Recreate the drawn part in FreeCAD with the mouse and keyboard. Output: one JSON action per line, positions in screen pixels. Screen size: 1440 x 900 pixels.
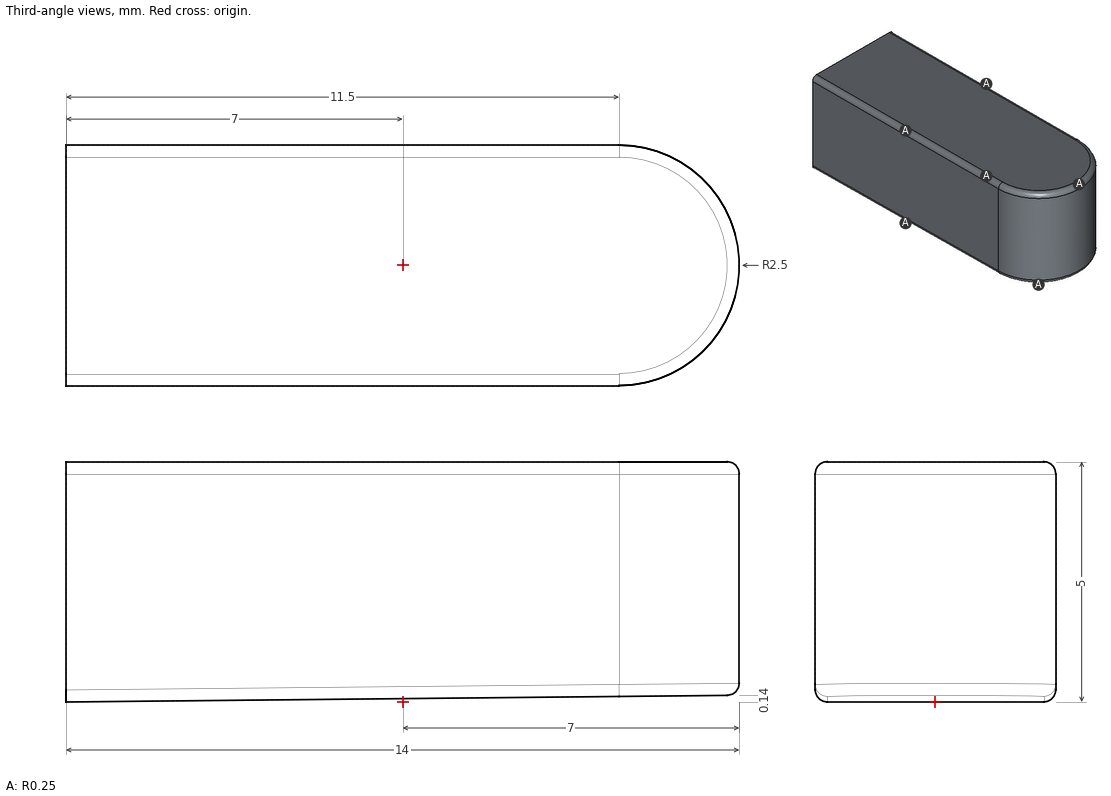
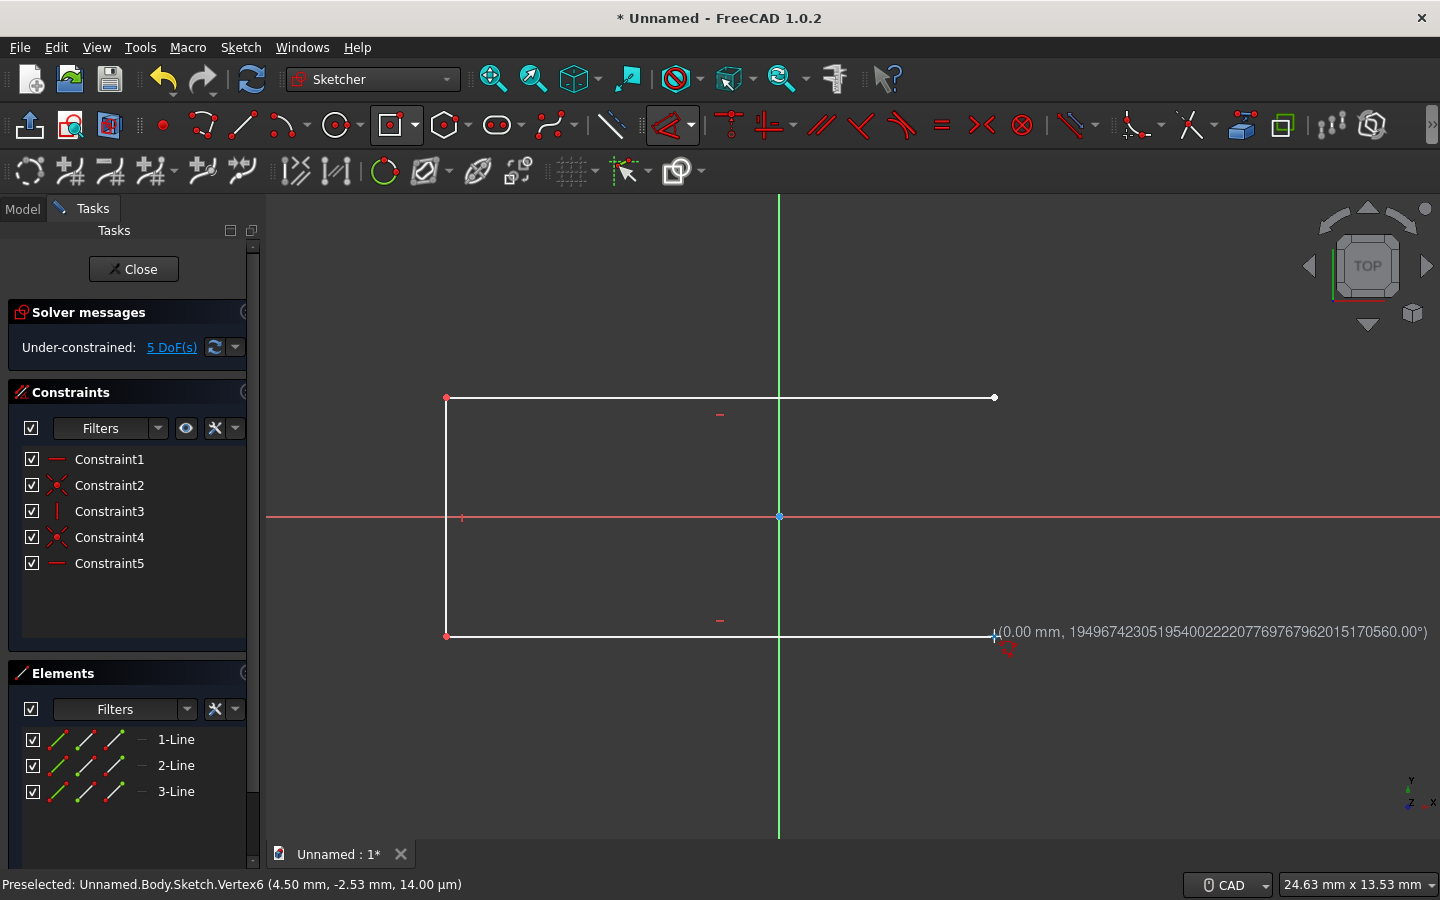
{"action": "key", "text": "g 3 a"}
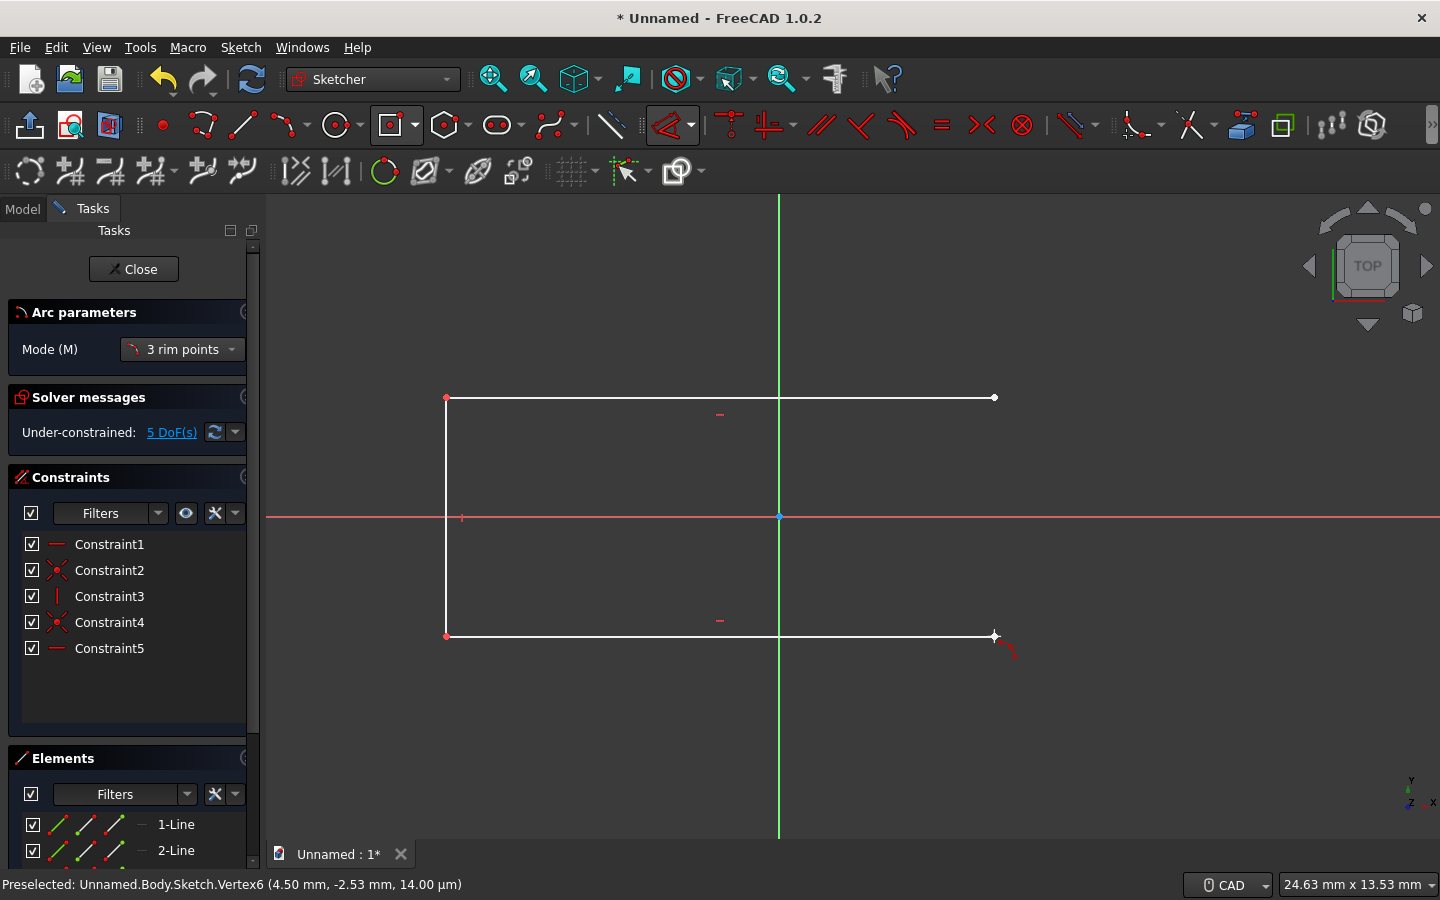
{"action": "left_click", "coordinate": [994, 637]}
{"action": "left_click", "coordinate": [994, 398]}
{"action": "left_click", "coordinate": [1107, 553]}
{"action": "key", "text": "Escape"}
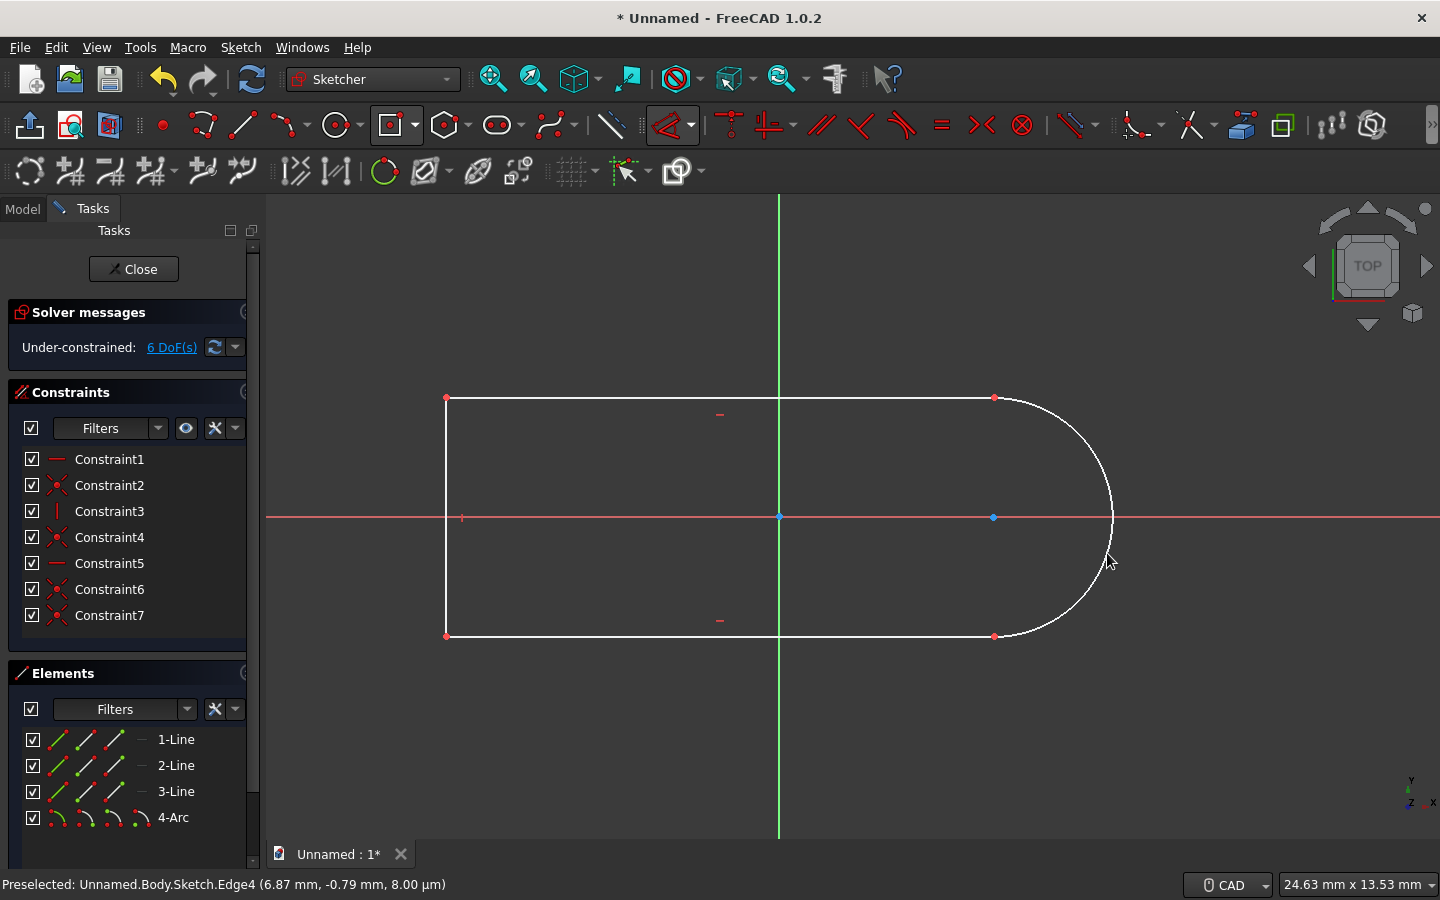
{"action": "left_click", "coordinate": [830, 398]}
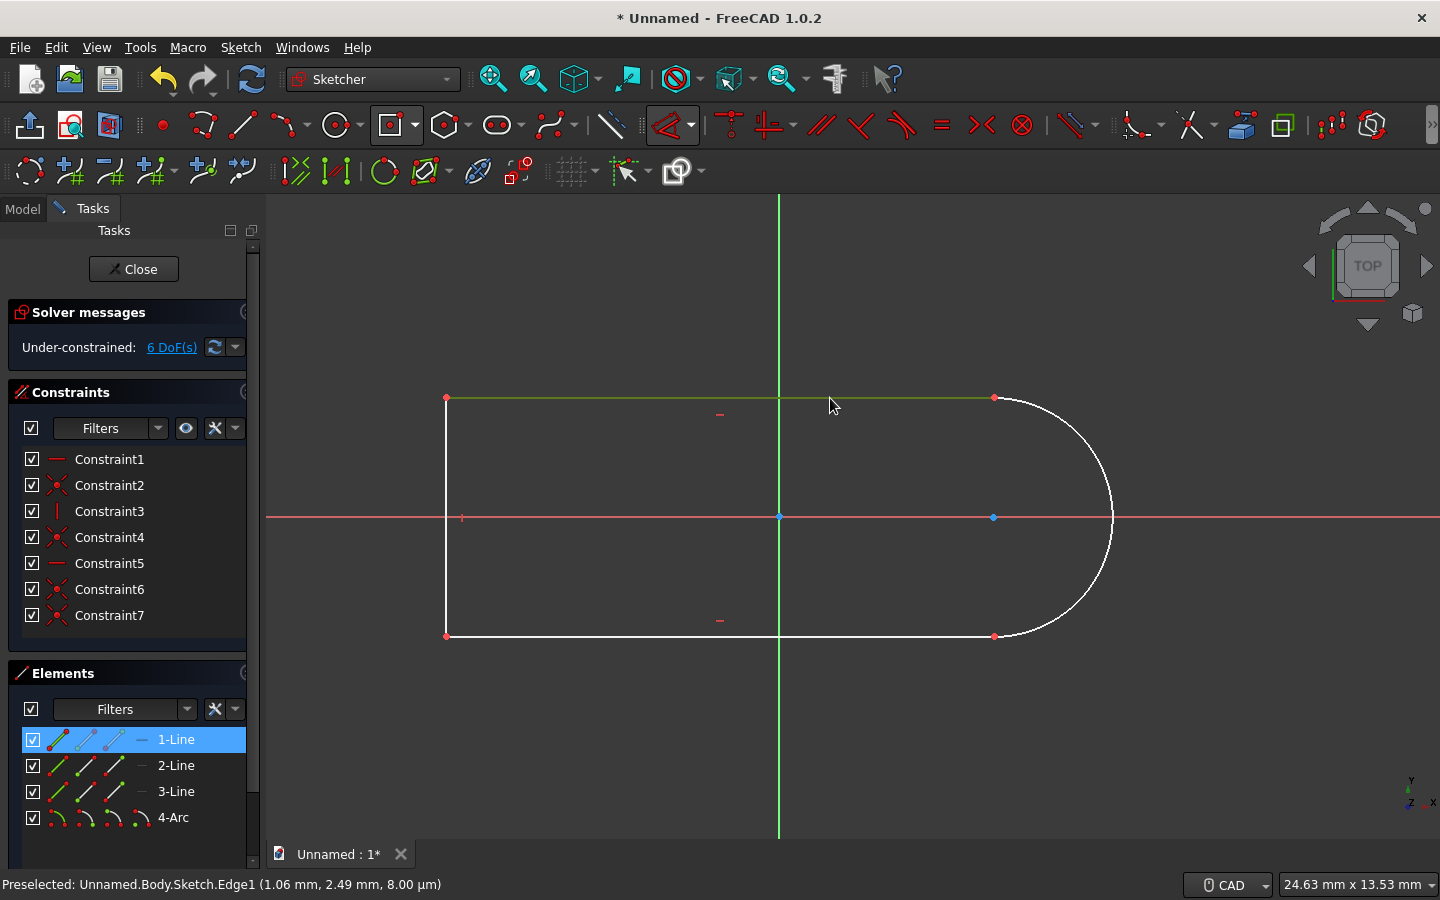
{"action": "left_click", "coordinate": [1090, 587]}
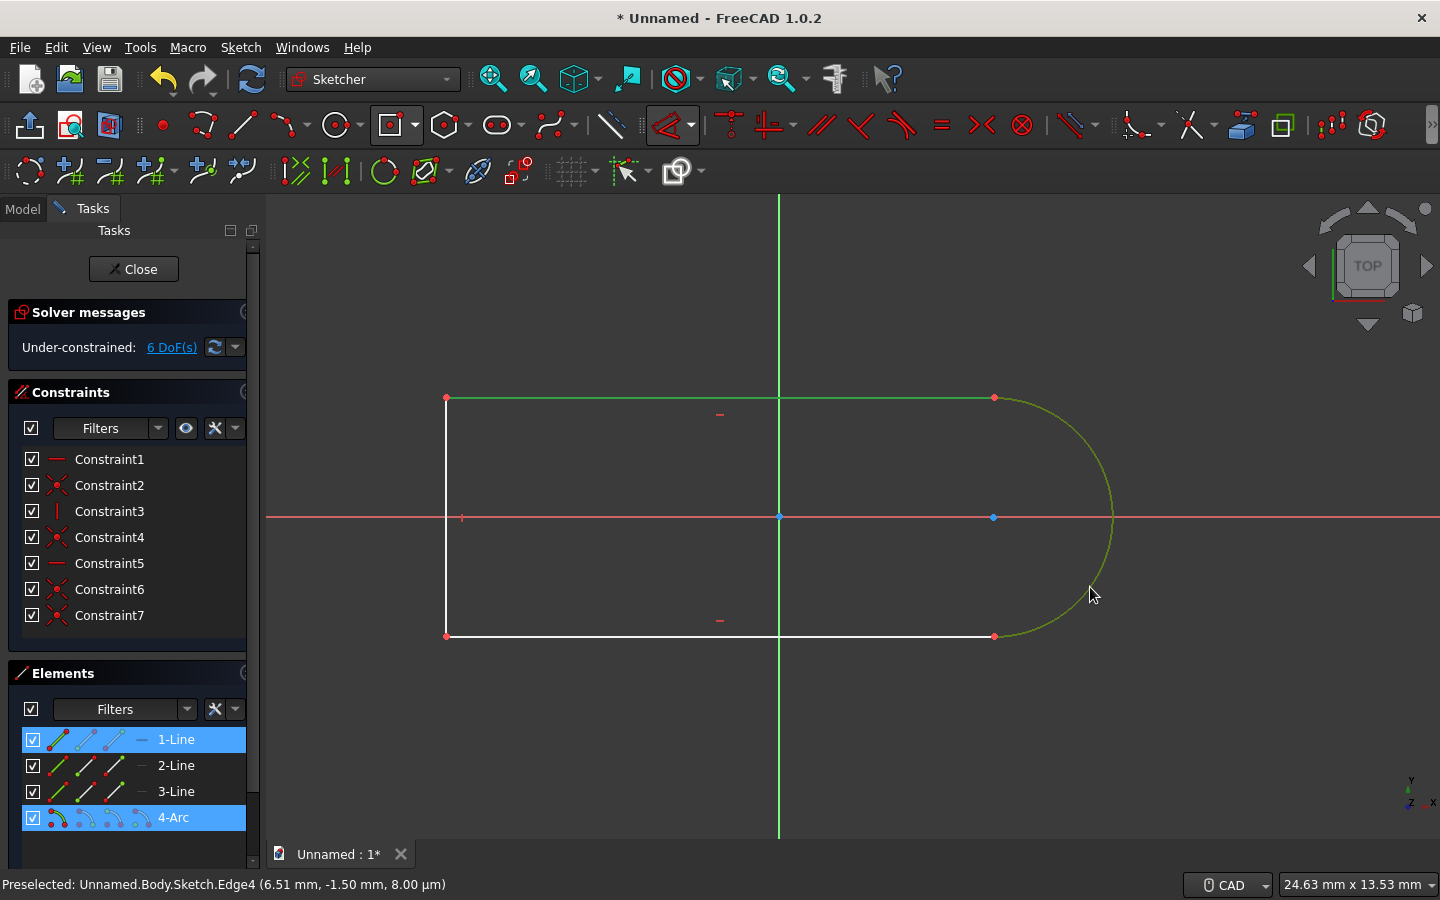
{"action": "key", "text": "t"}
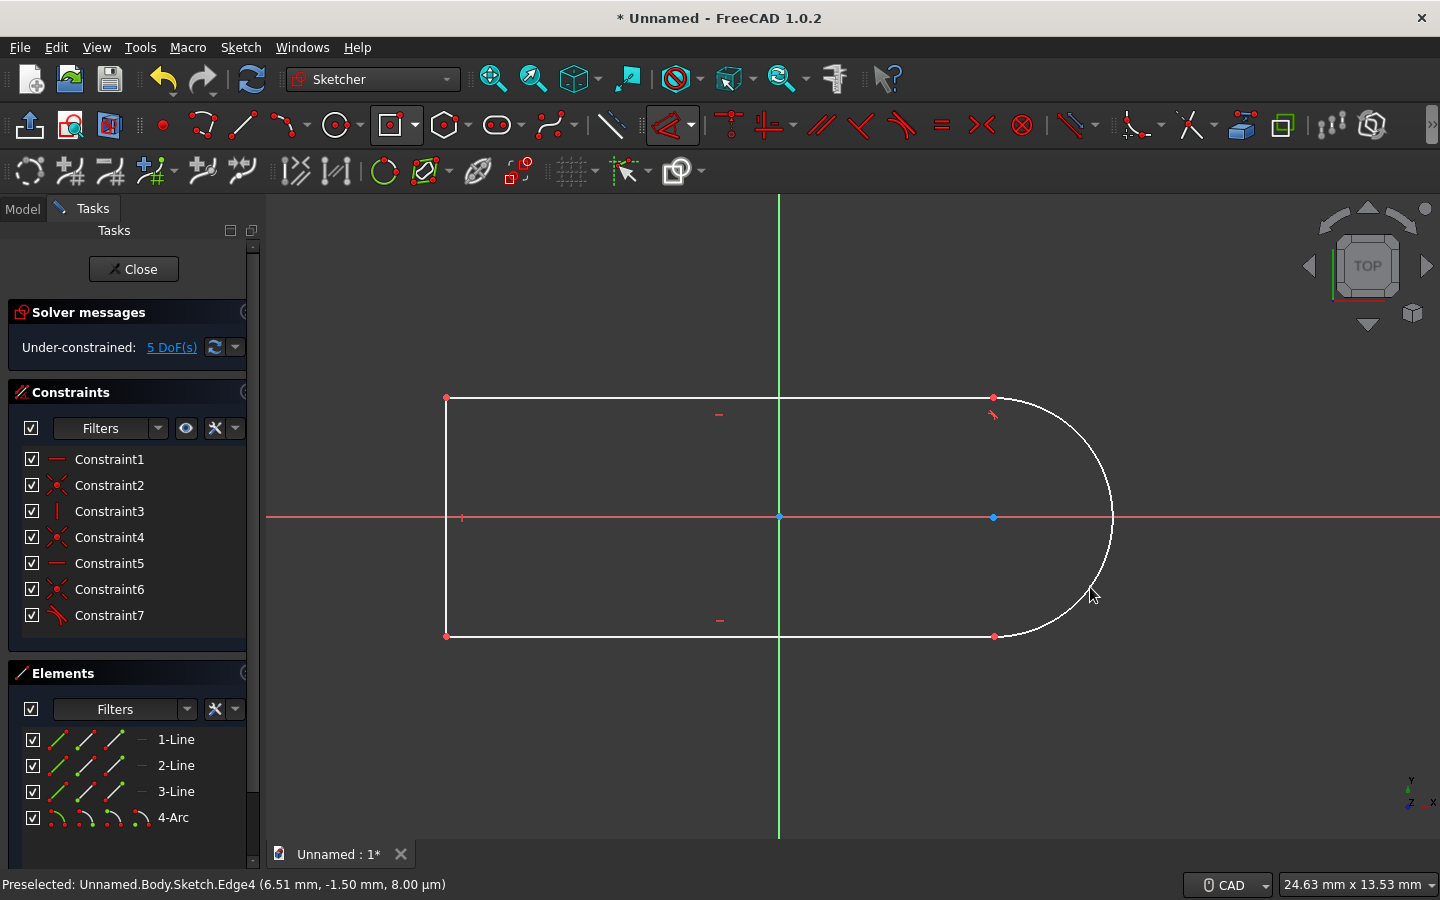
{"action": "left_click", "coordinate": [610, 637]}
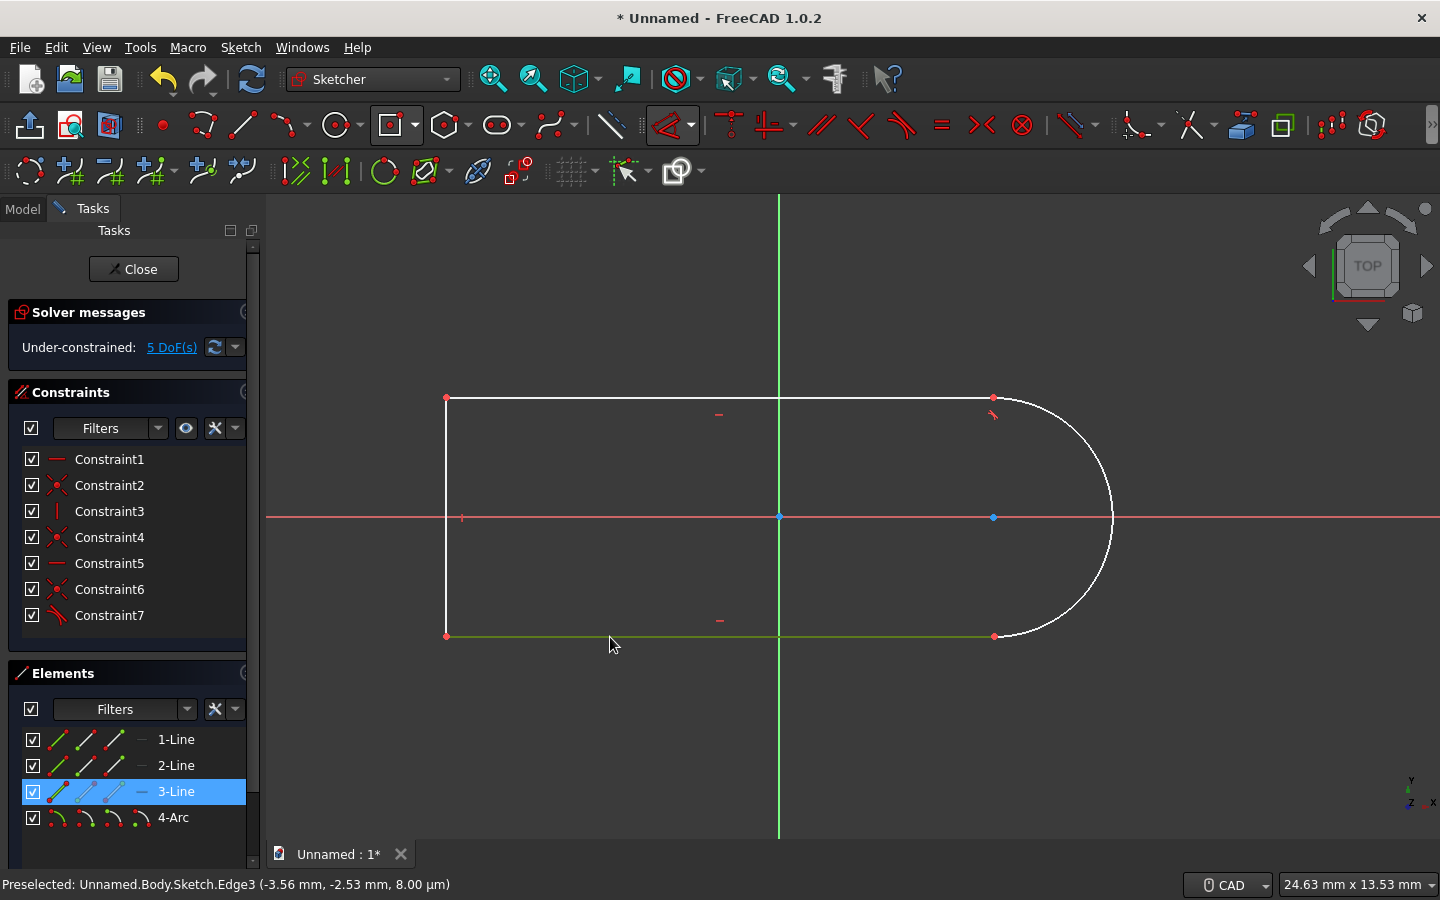
{"action": "left_click", "coordinate": [1090, 587]}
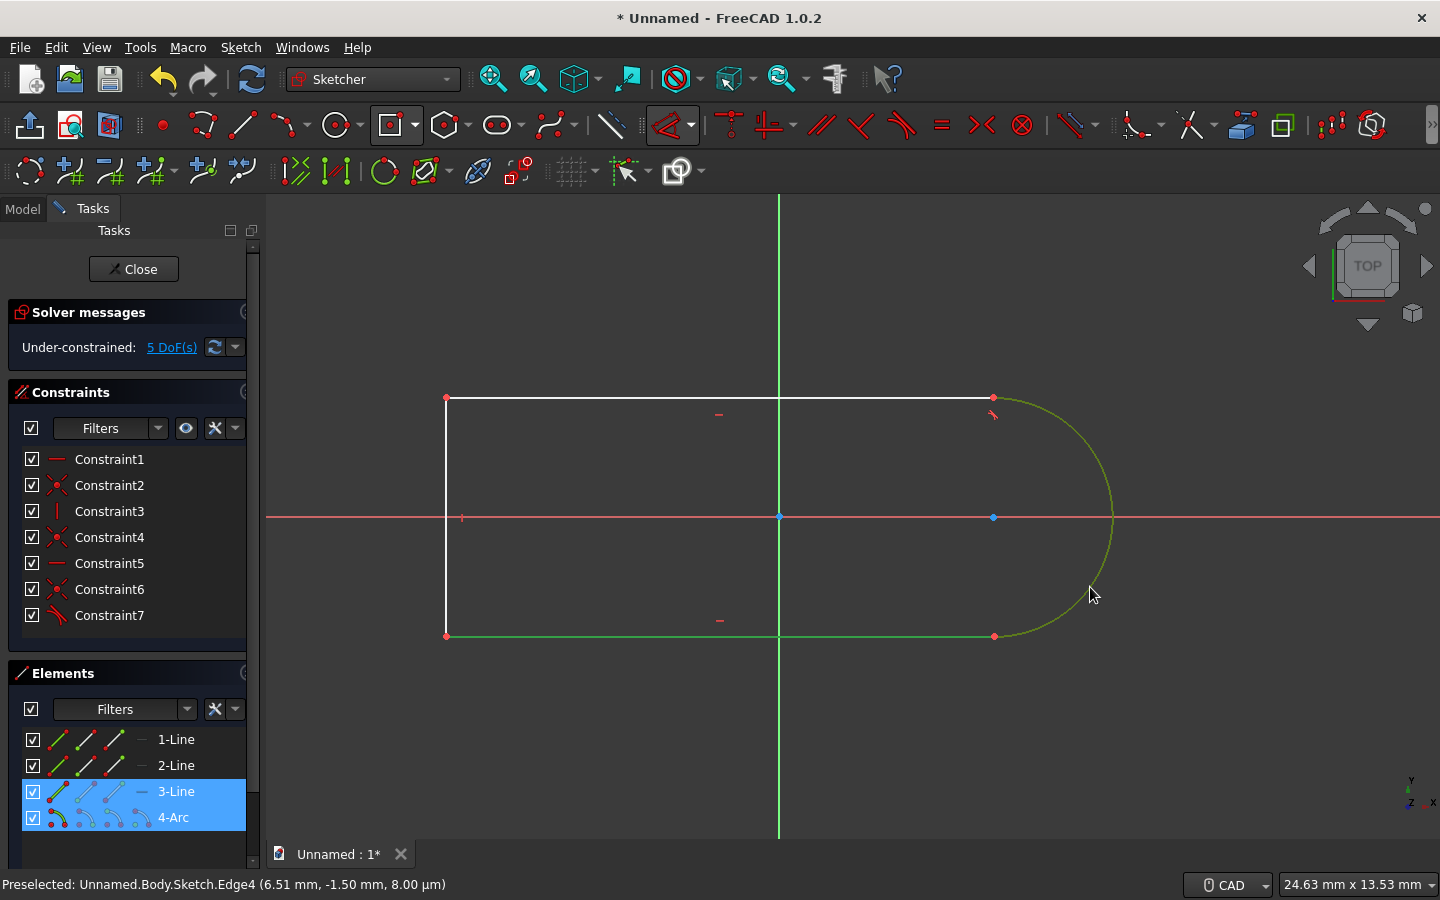
{"action": "key", "text": "t"}